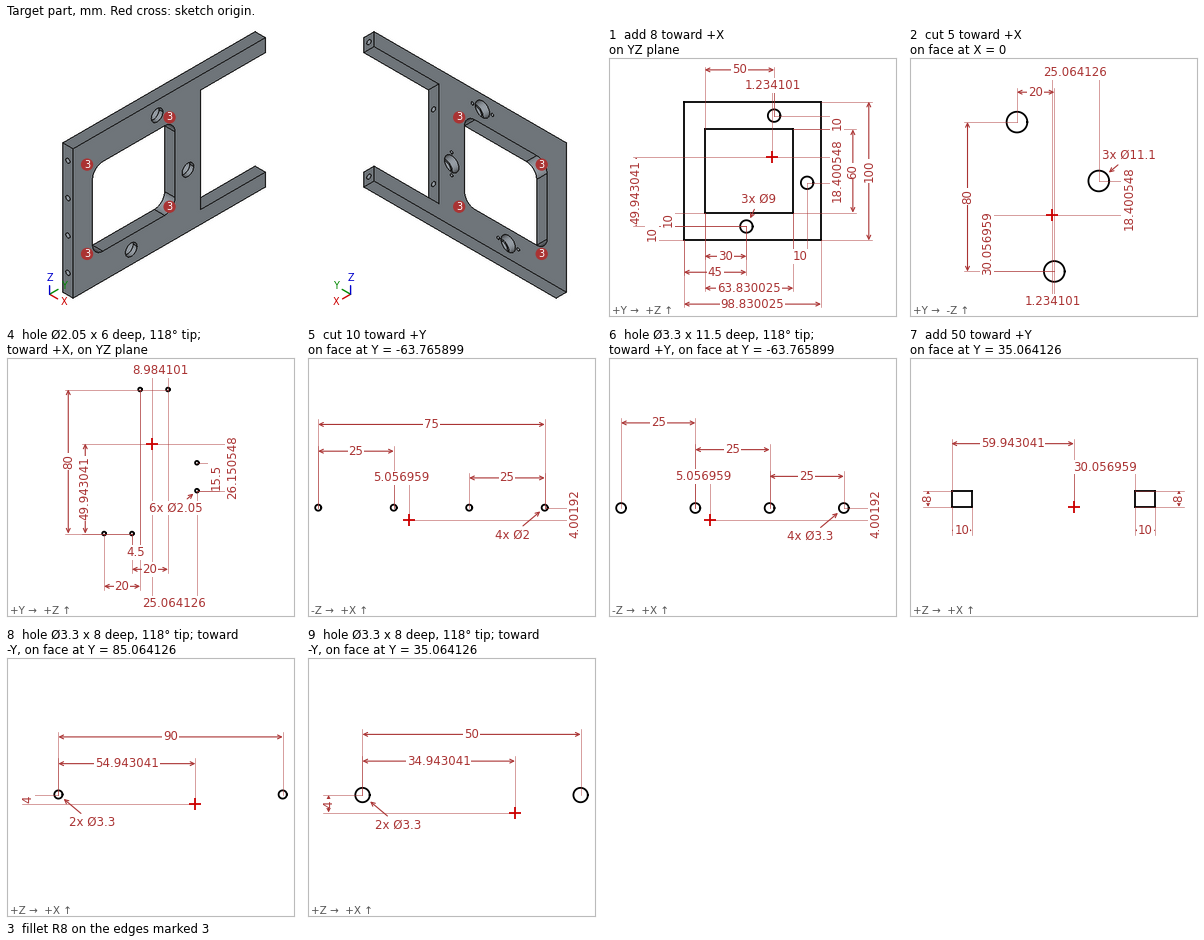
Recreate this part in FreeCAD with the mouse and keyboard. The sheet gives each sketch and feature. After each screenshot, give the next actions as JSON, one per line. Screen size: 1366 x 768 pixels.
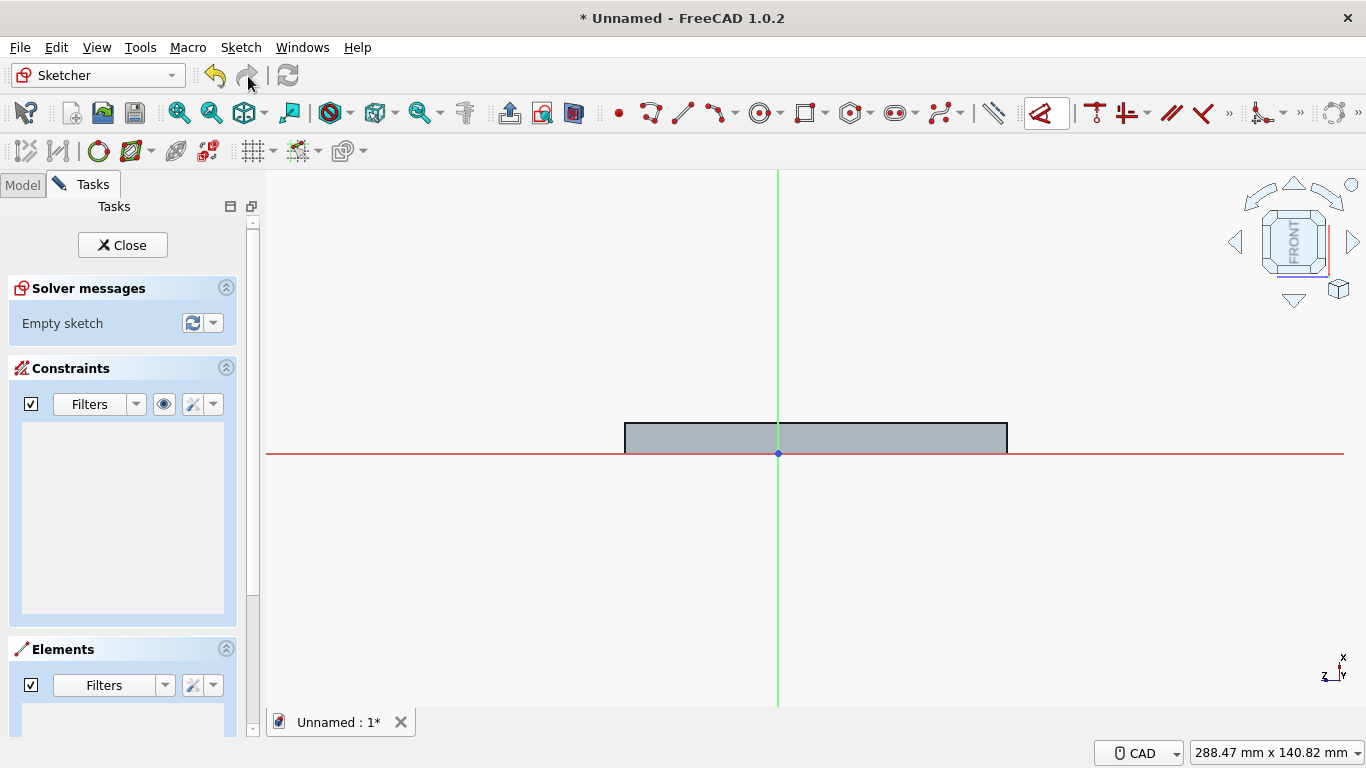
{"action": "scroll", "coordinate": [855, 449], "scroll_direction": "up", "scroll_amount": 4}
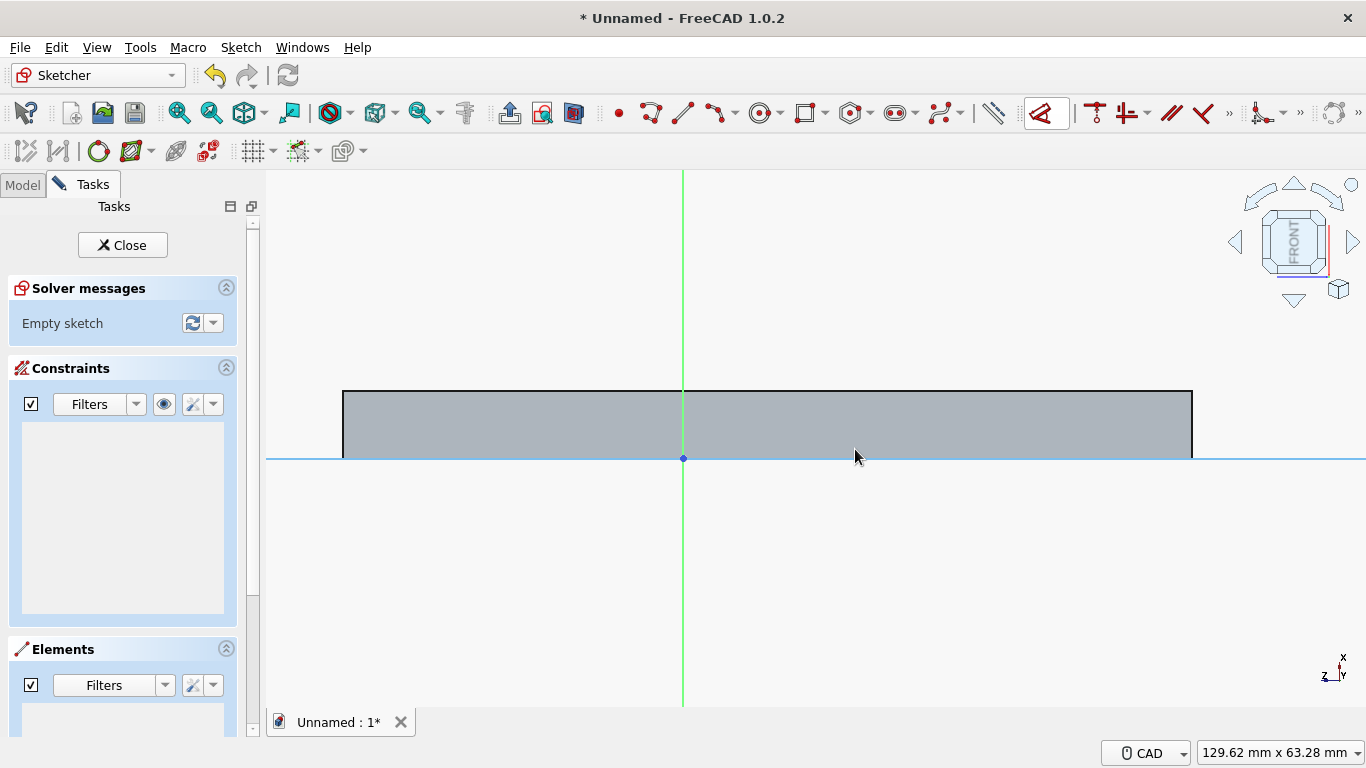
{"action": "left_click", "coordinate": [760, 114]}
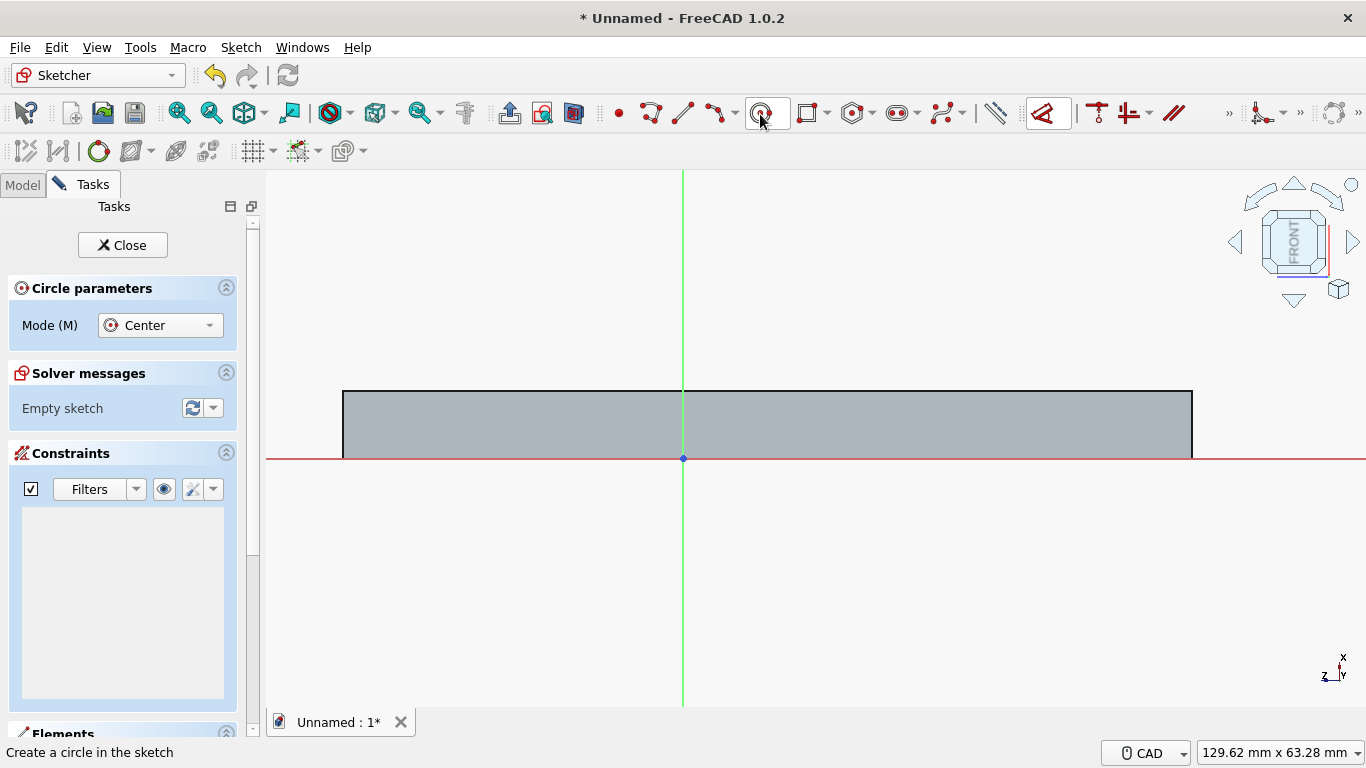
{"action": "scroll", "coordinate": [1065, 425], "scroll_direction": "up", "scroll_amount": 5}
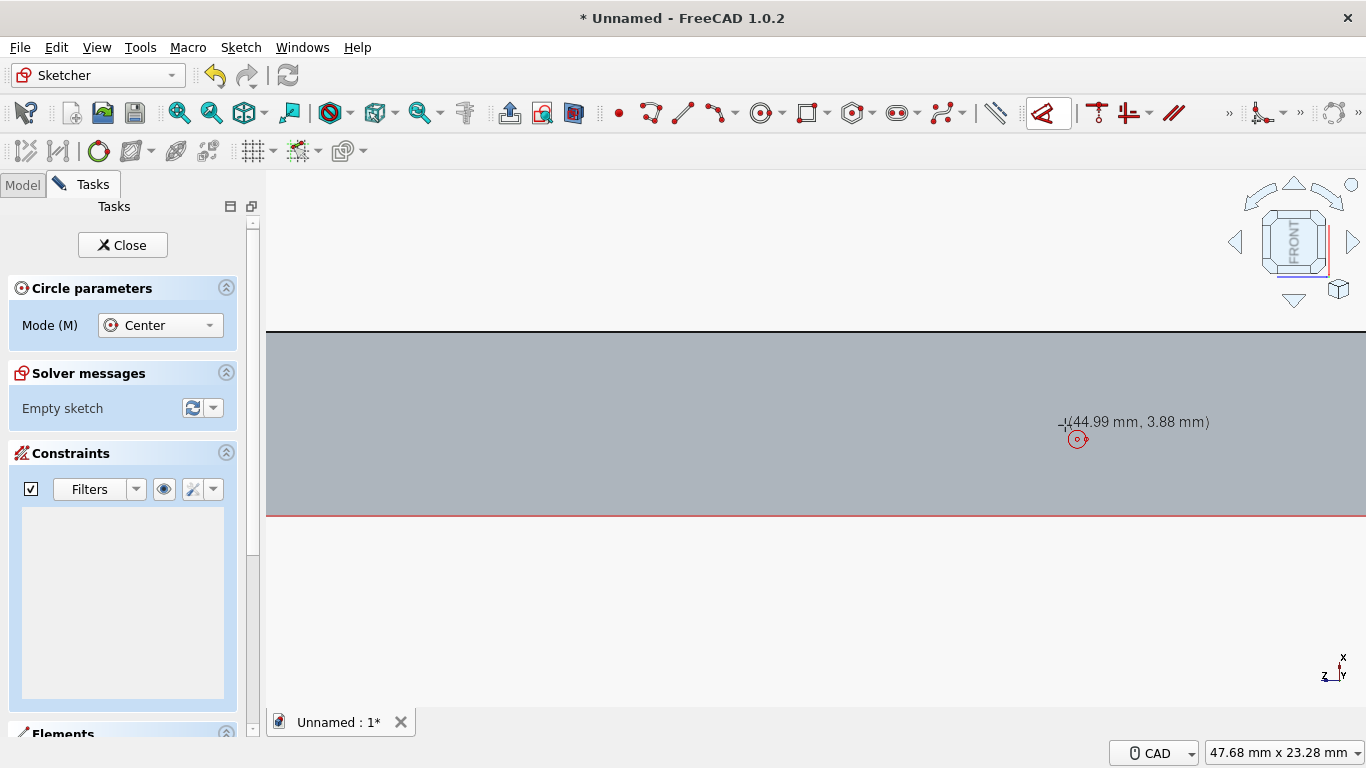
{"action": "left_click", "coordinate": [1063, 424]}
{"action": "mouse_move", "coordinate": [1079, 408]}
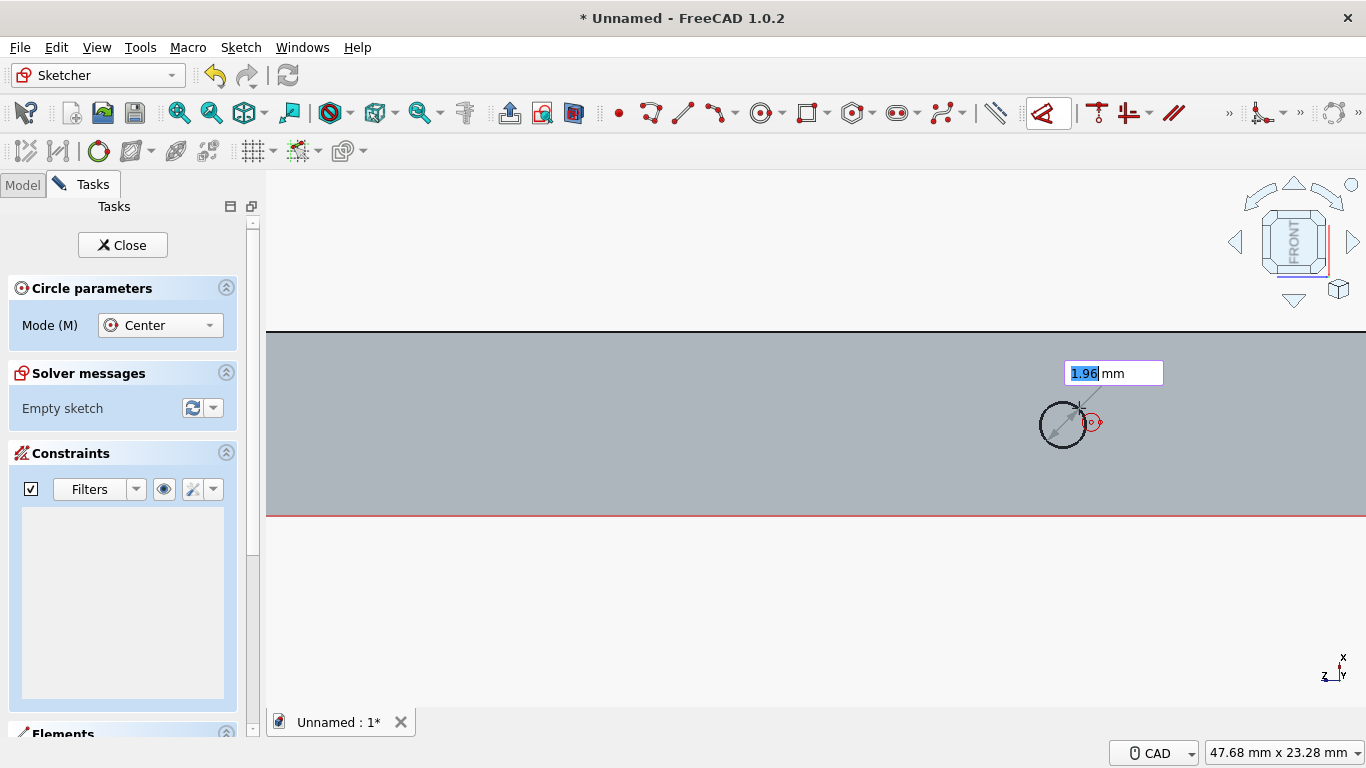
{"action": "type", "text": "2"}
{"action": "key", "text": "Return"}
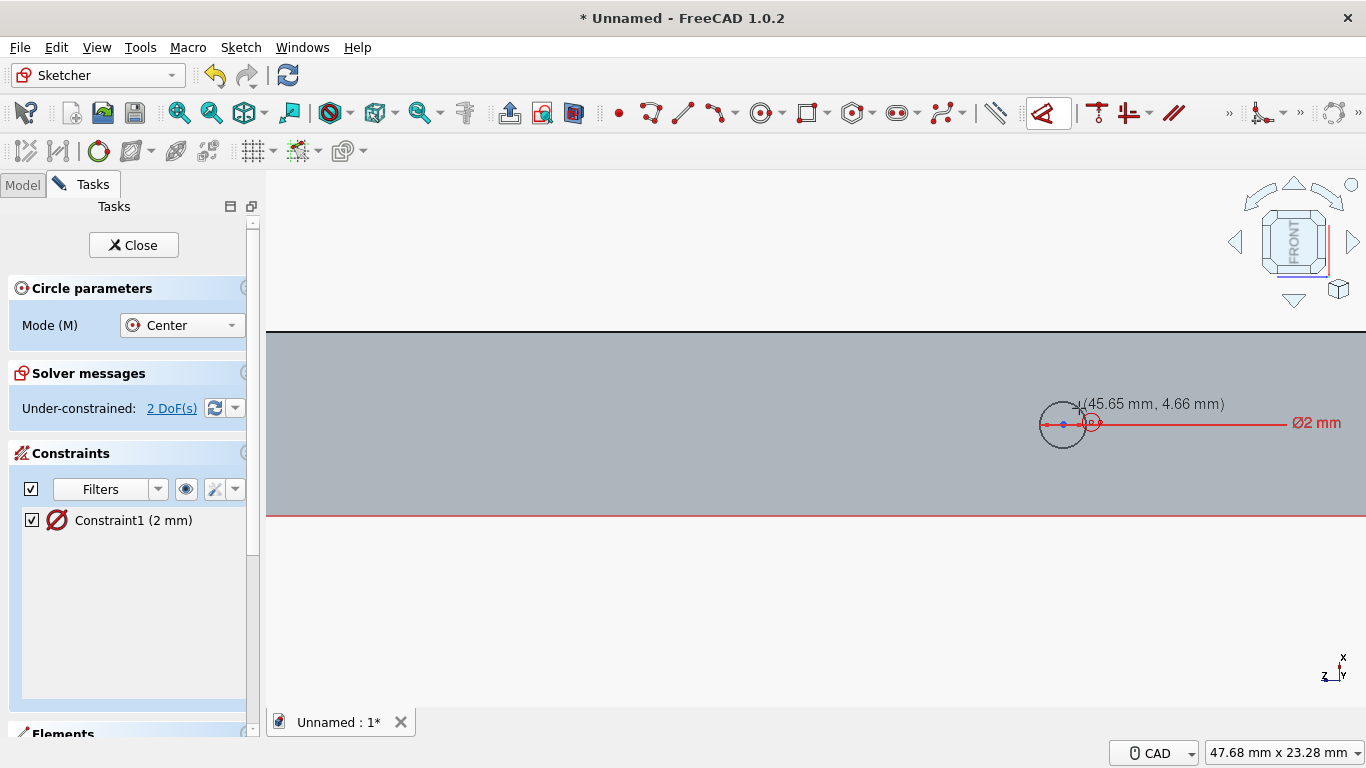
{"action": "scroll", "coordinate": [1068, 427], "scroll_direction": "down", "scroll_amount": 5}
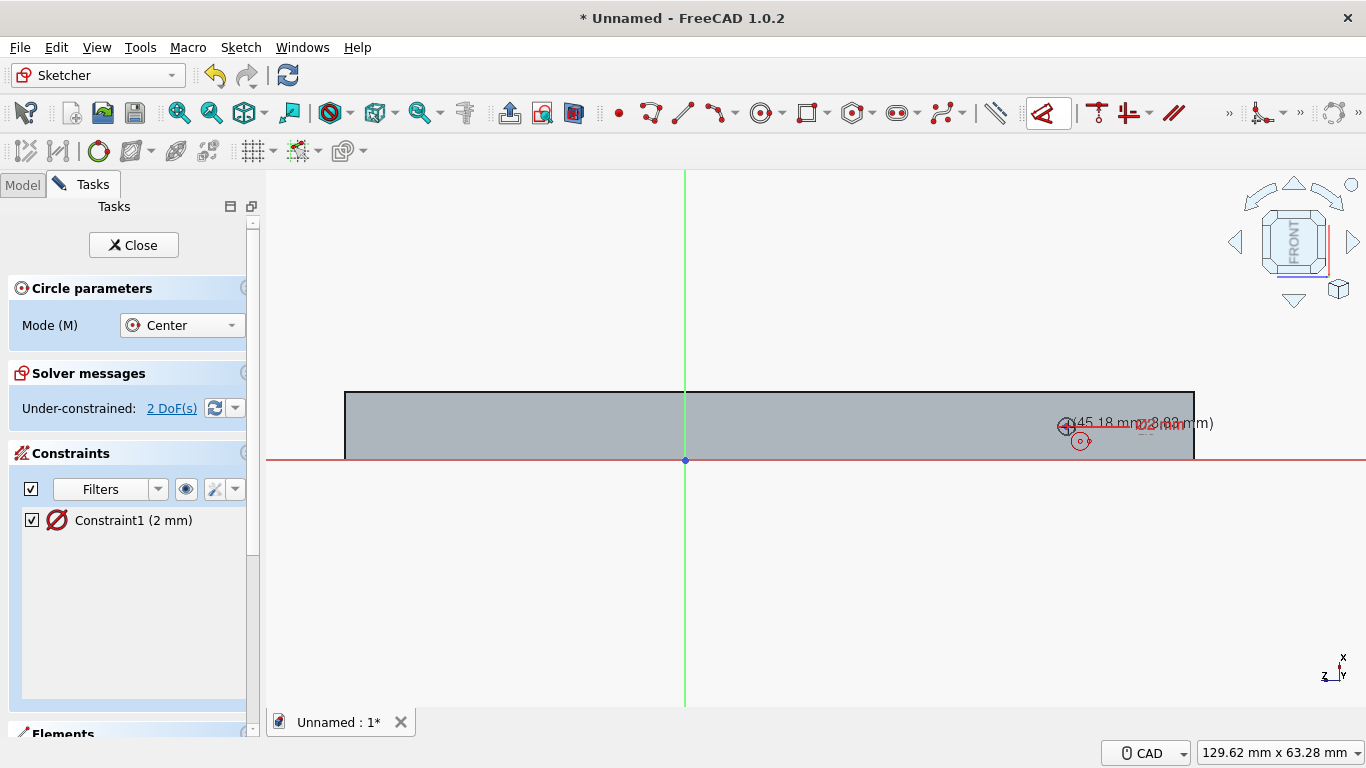
{"action": "scroll", "coordinate": [430, 426], "scroll_direction": "up", "scroll_amount": 5}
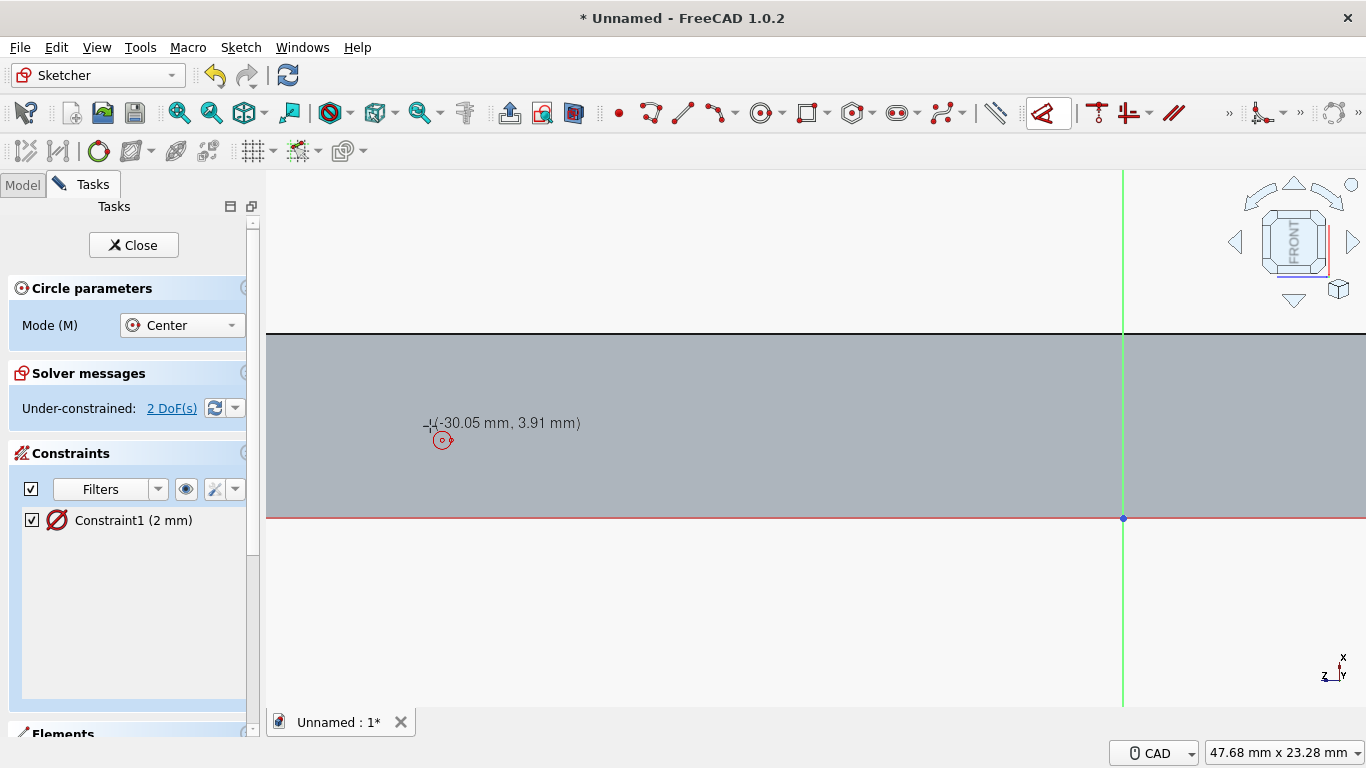
{"action": "left_click", "coordinate": [430, 426]}
{"action": "mouse_move", "coordinate": [446, 410]}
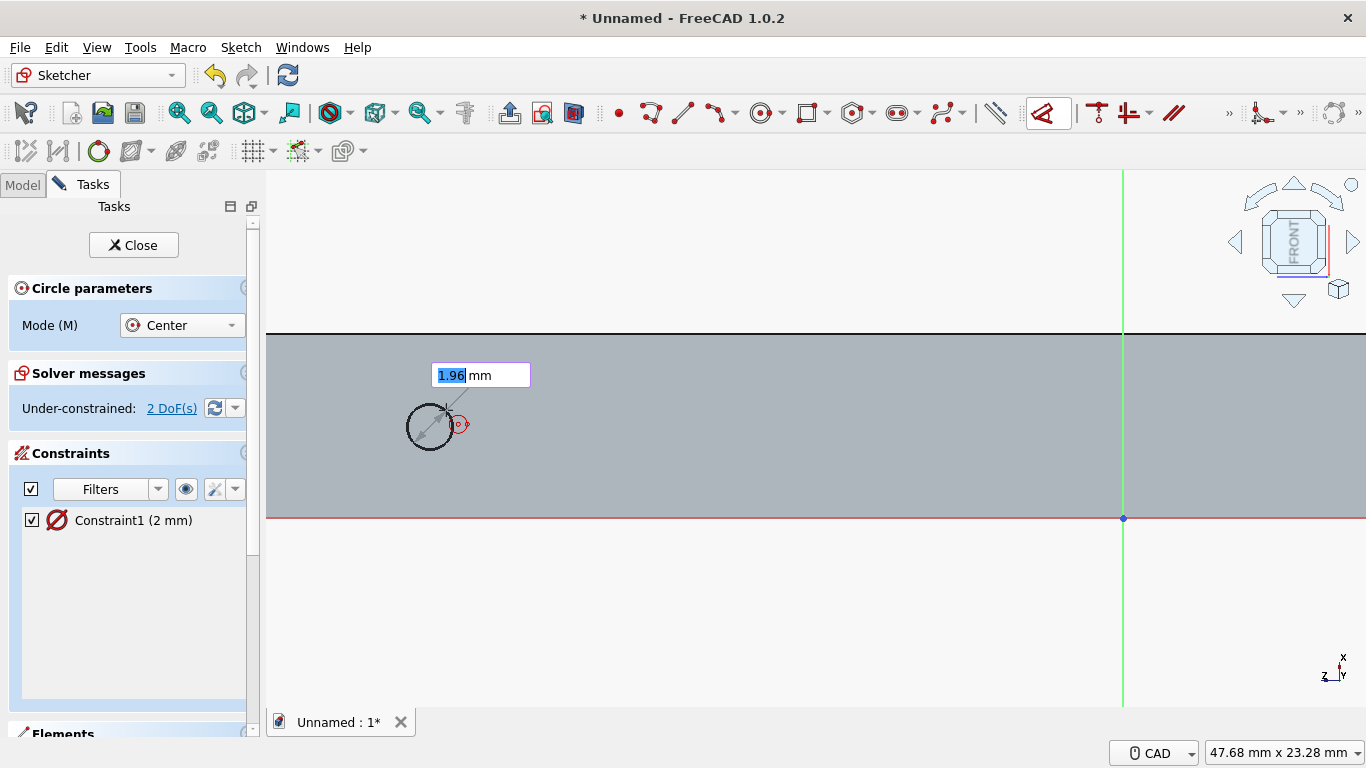
{"action": "type", "text": "2"}
{"action": "key", "text": "Return"}